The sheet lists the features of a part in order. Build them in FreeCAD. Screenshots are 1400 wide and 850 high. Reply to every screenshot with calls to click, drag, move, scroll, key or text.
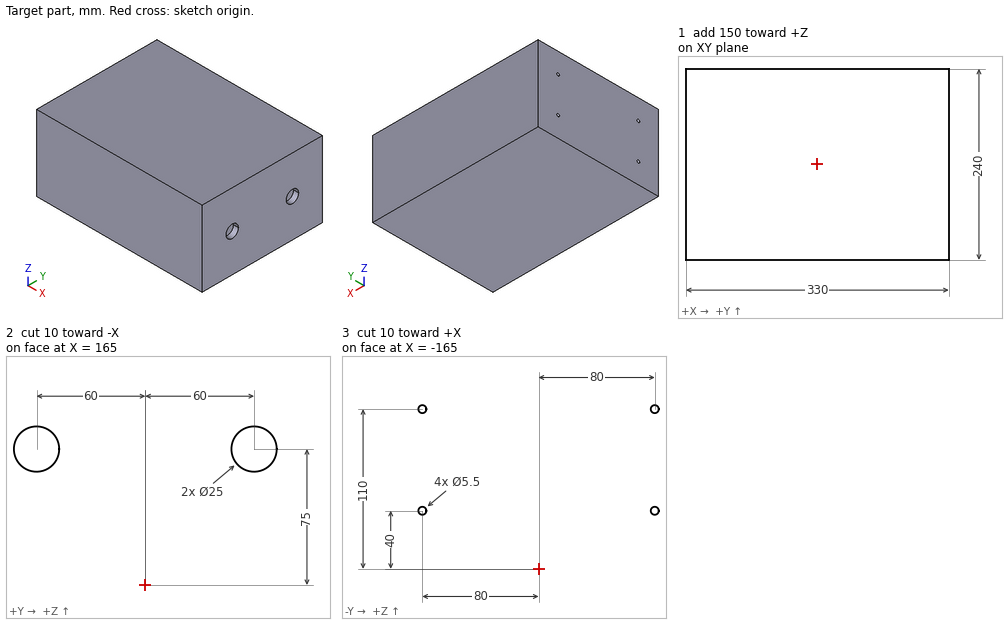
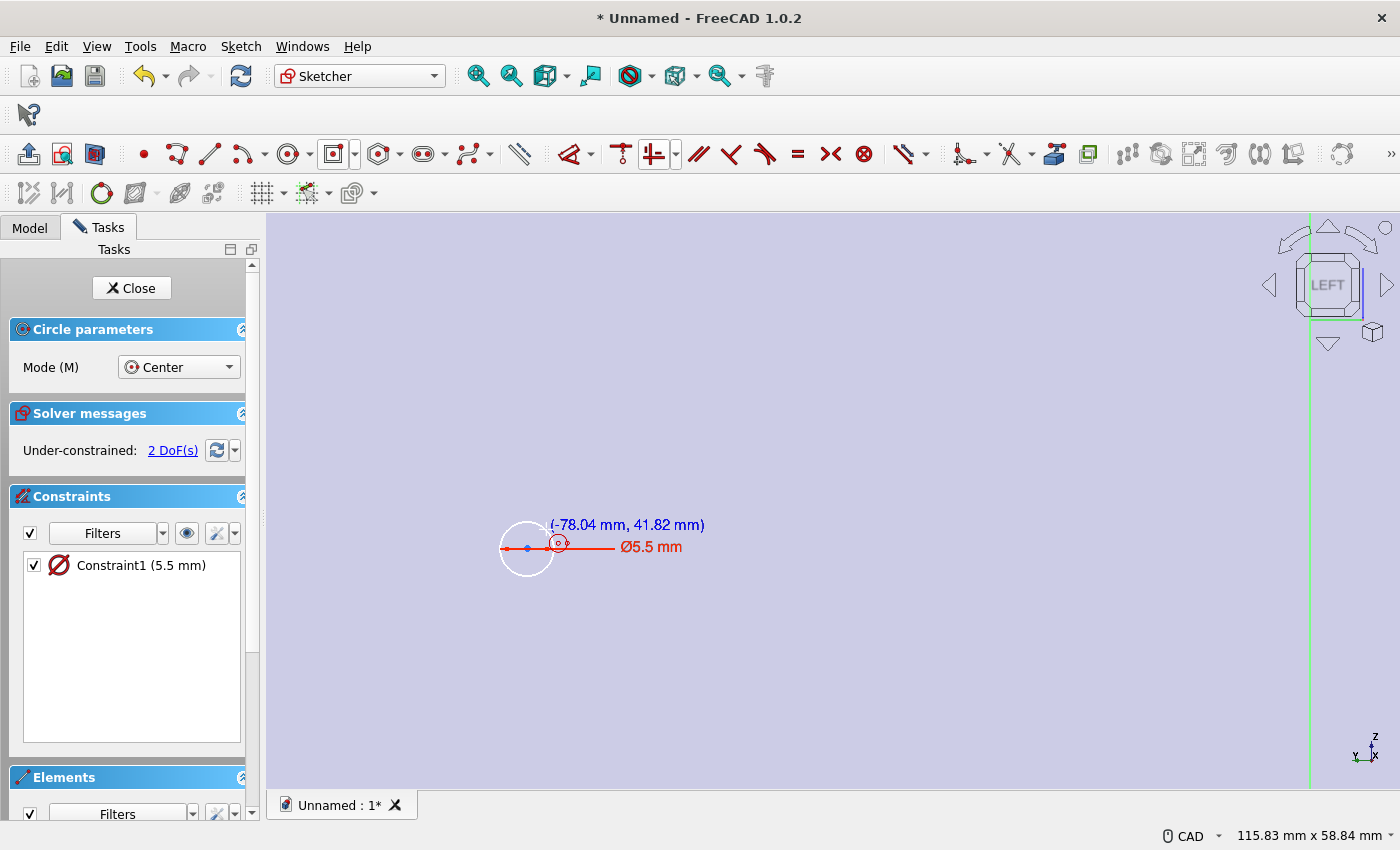
scroll(529, 550, down, 6)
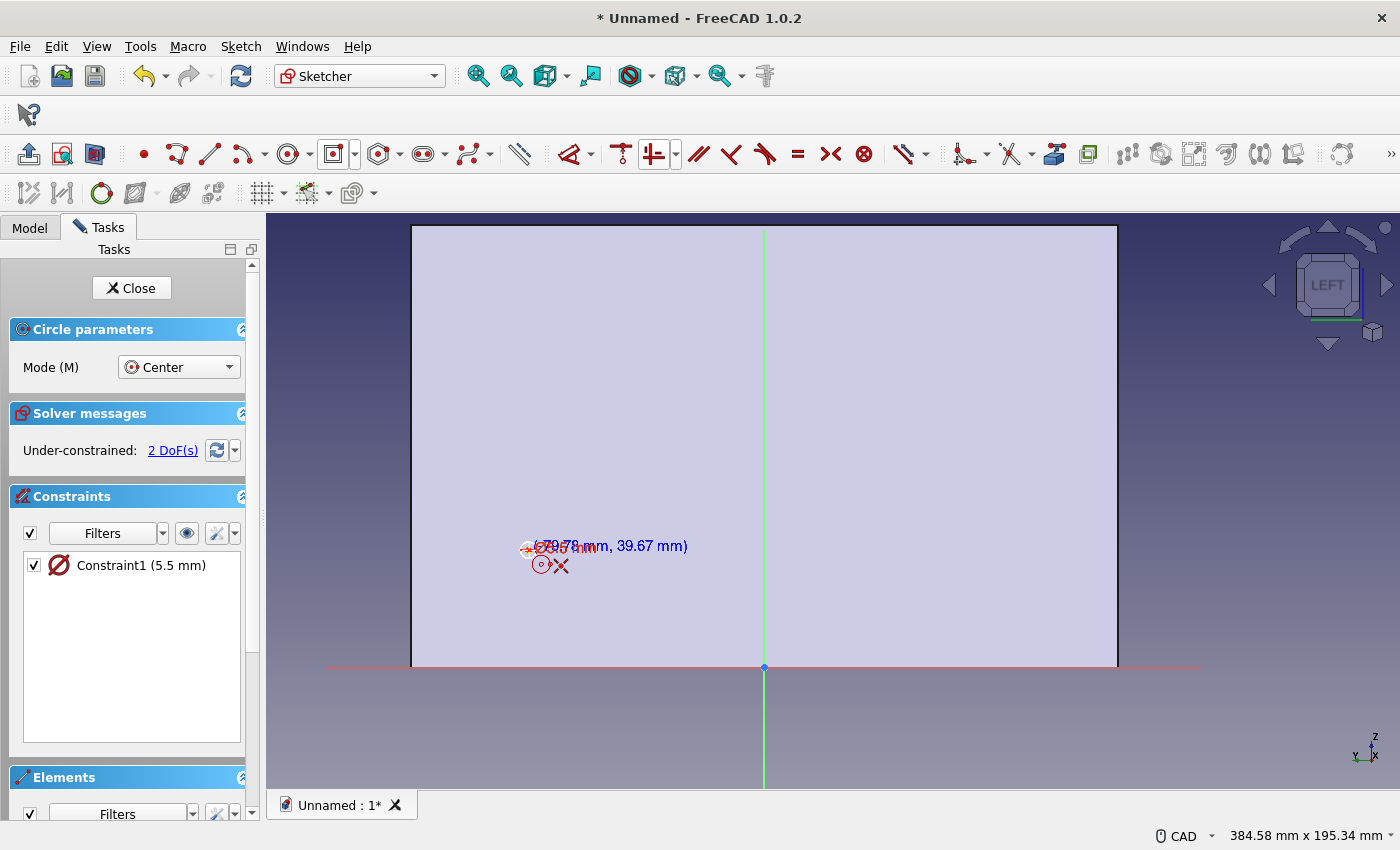
scroll(529, 343, up, 6)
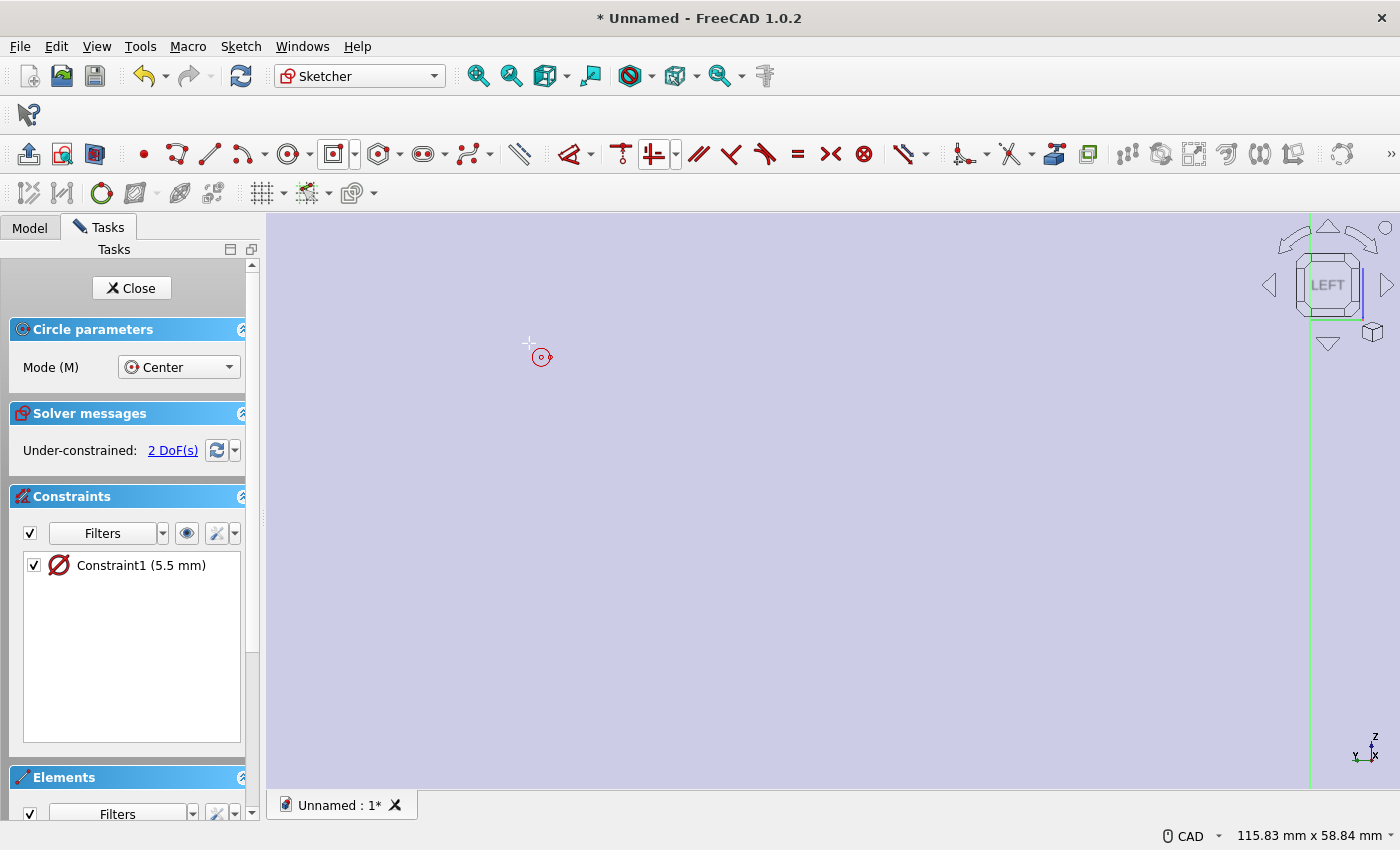
click(527, 344)
move(546, 325)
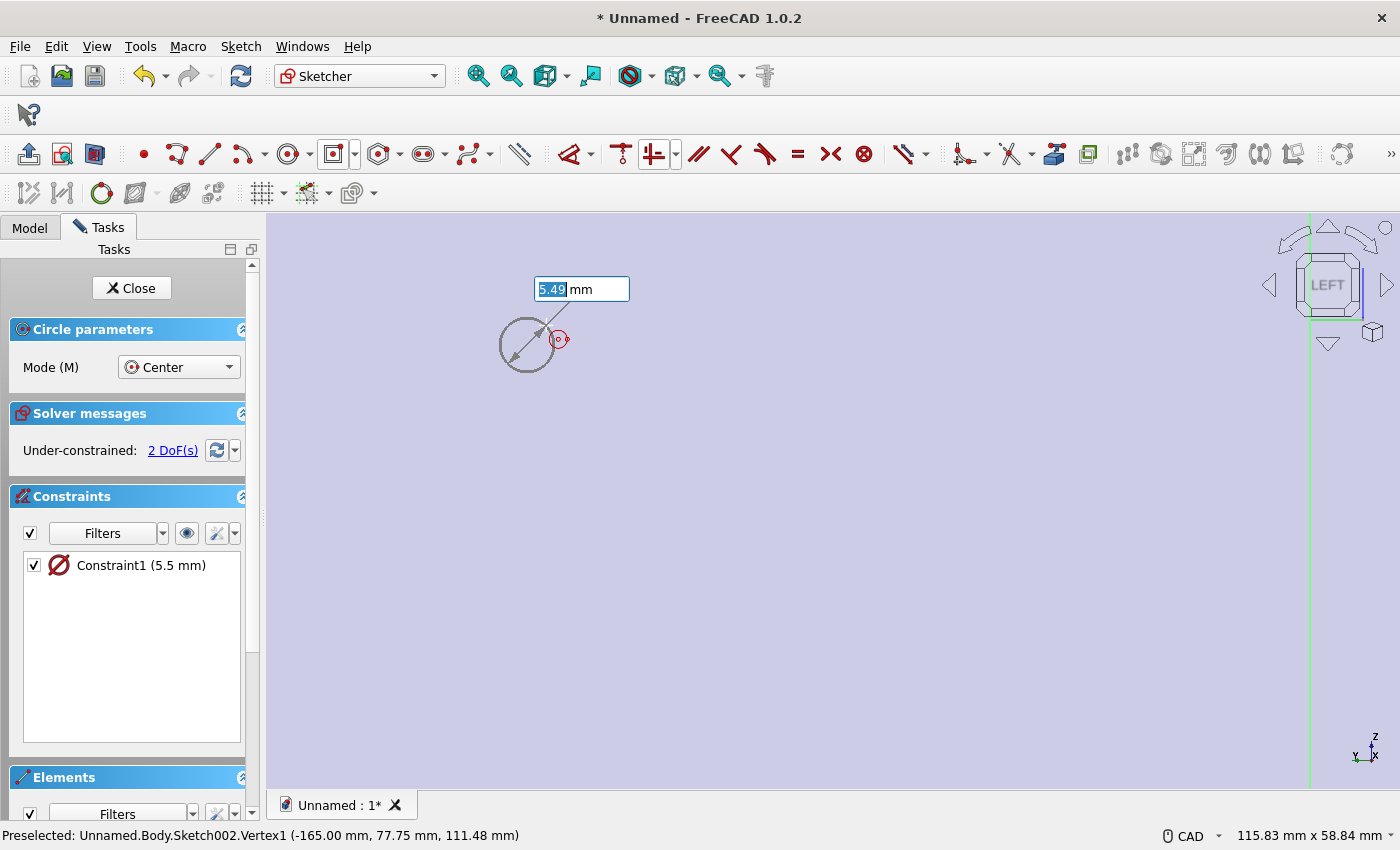
text(5.5)
key(Return)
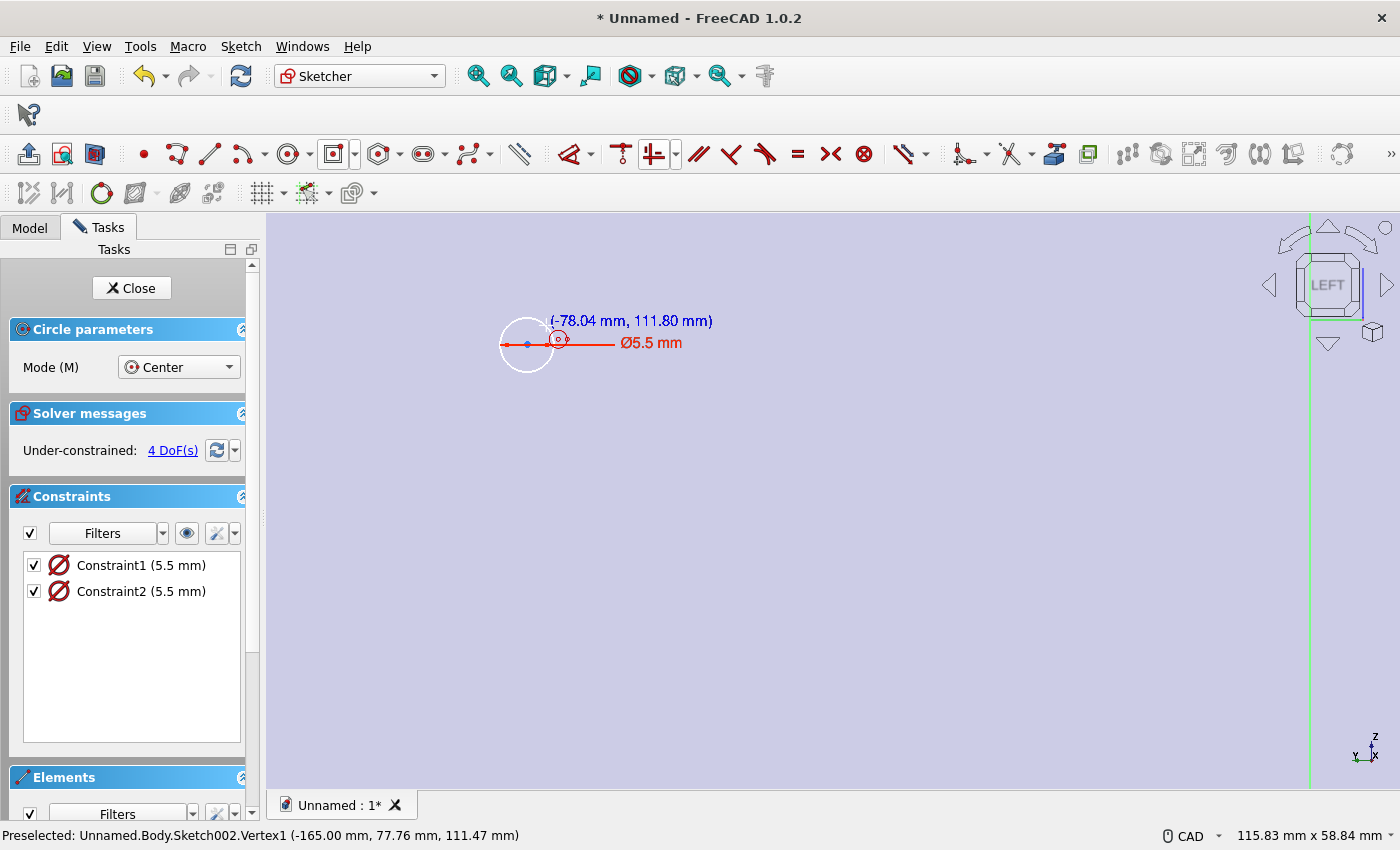
scroll(529, 343, down, 6)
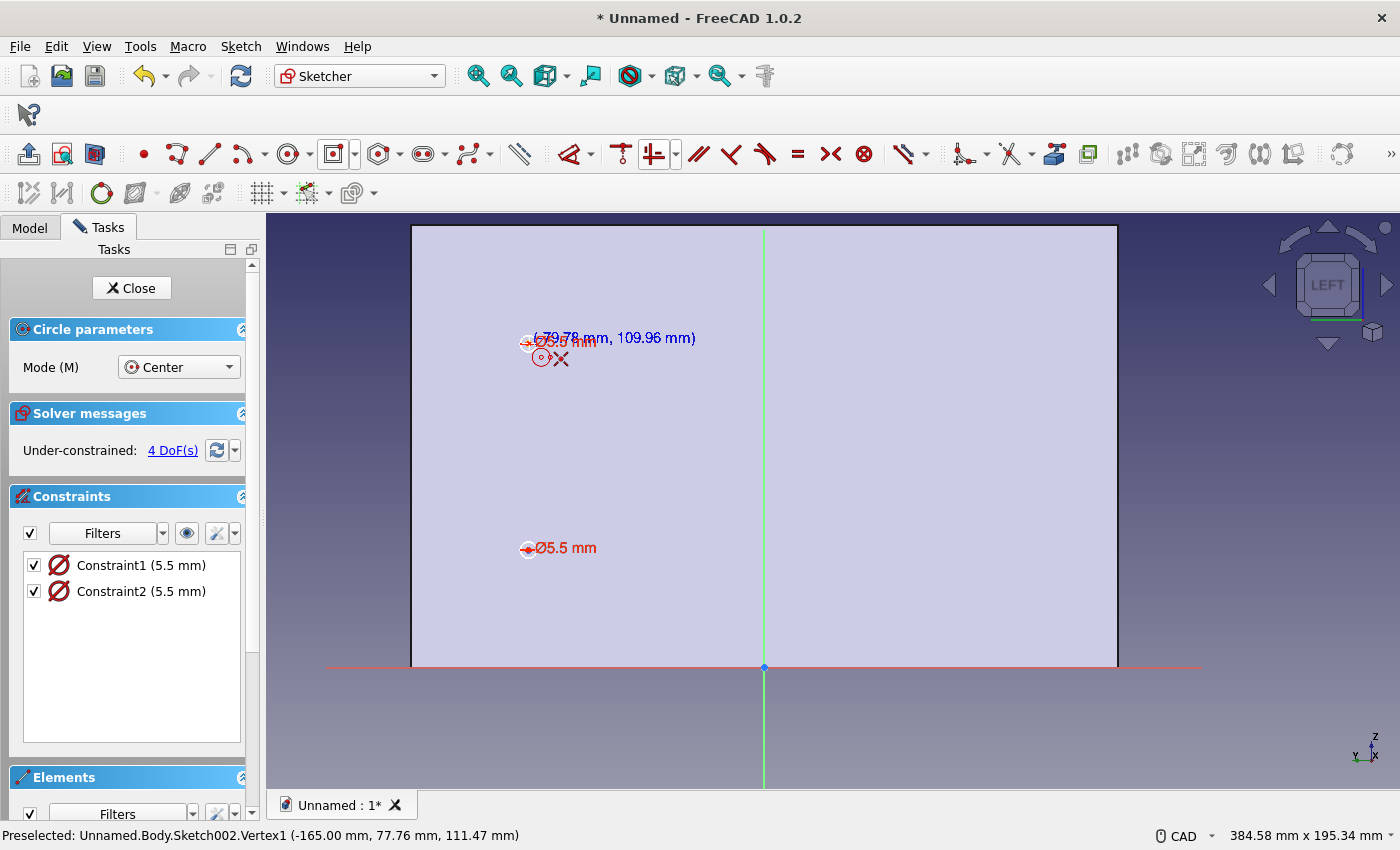
scroll(1000, 343, up, 6)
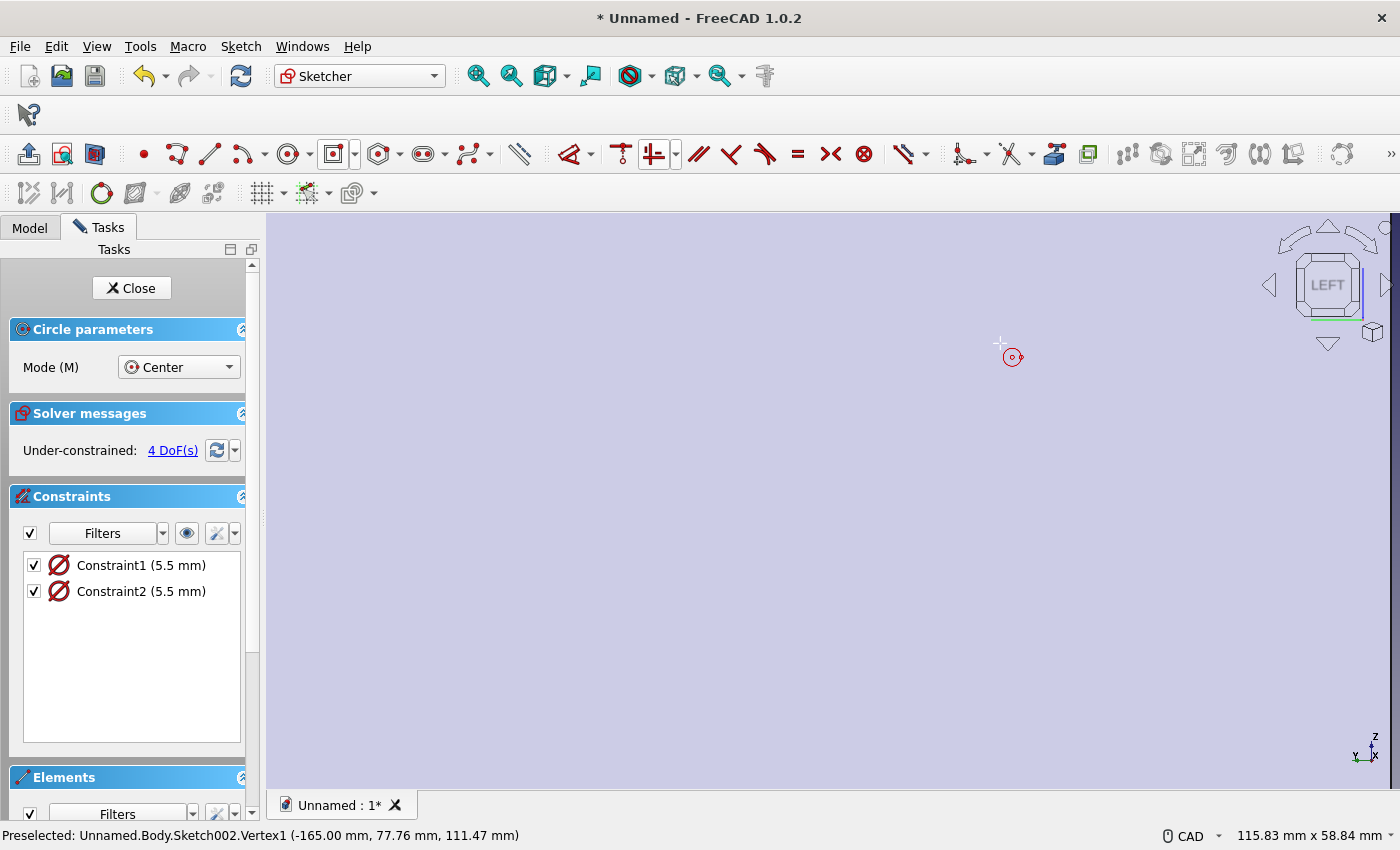
click(999, 344)
move(1018, 325)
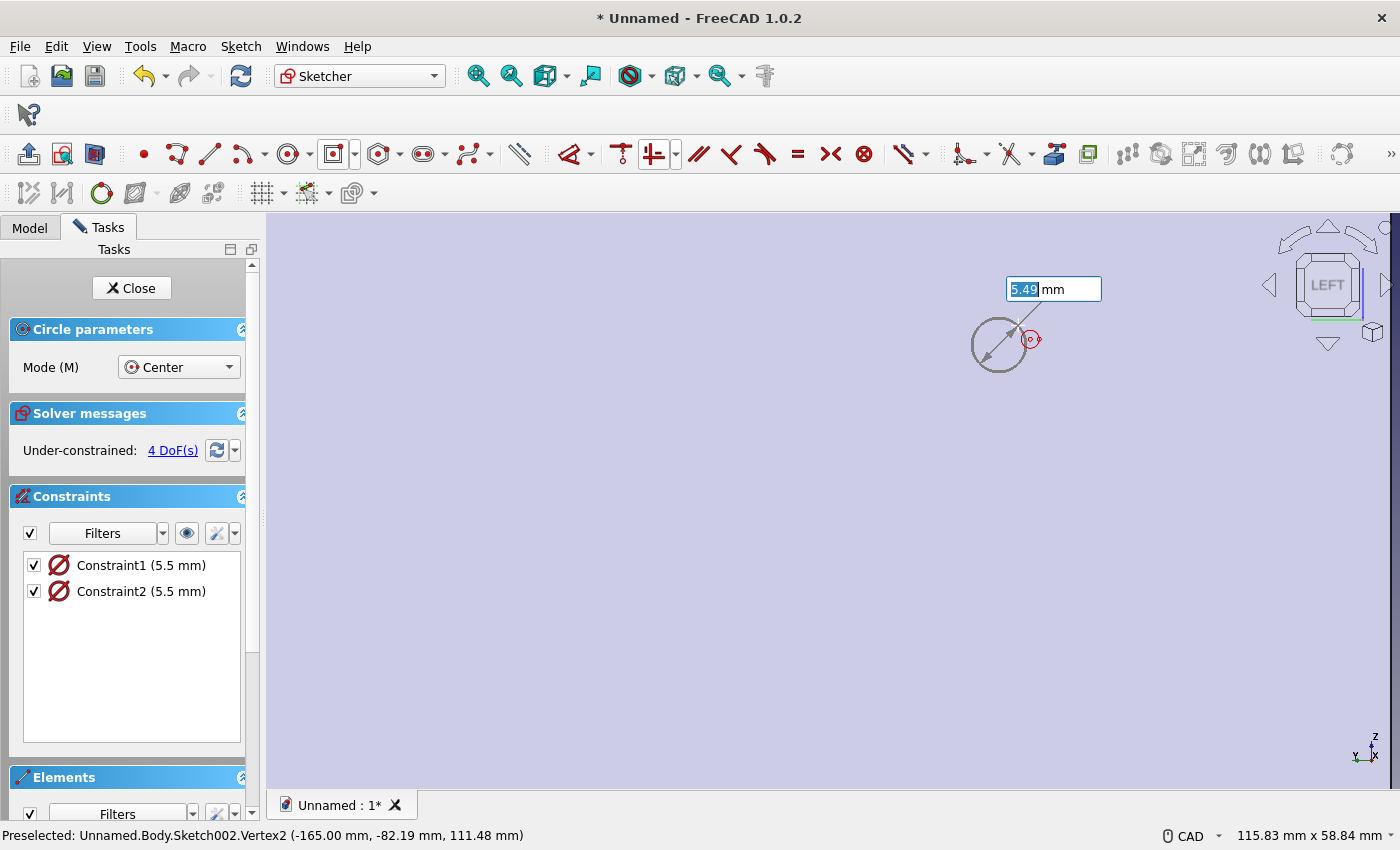
text(5.5)
key(Return)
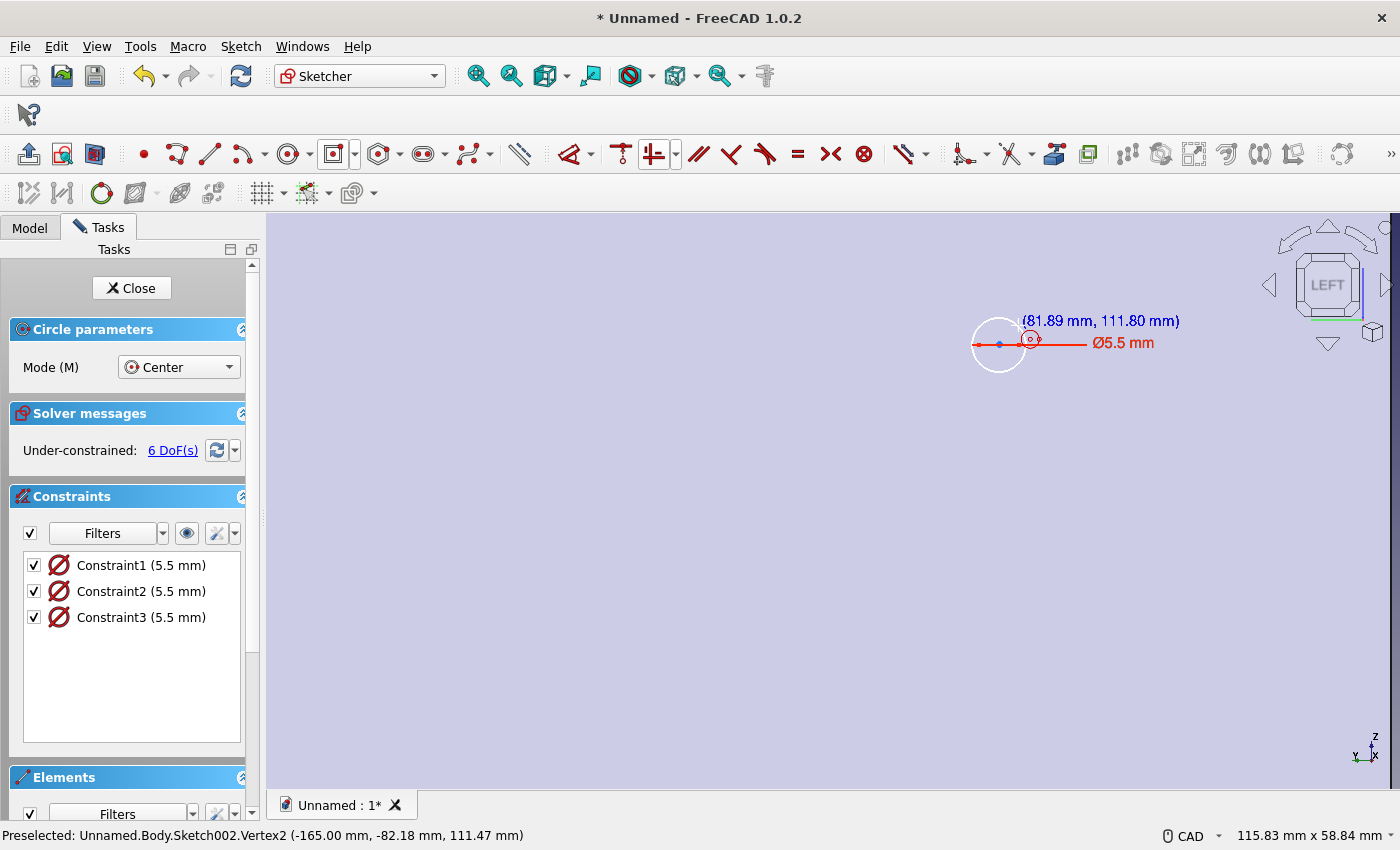
scroll(1001, 343, down, 6)